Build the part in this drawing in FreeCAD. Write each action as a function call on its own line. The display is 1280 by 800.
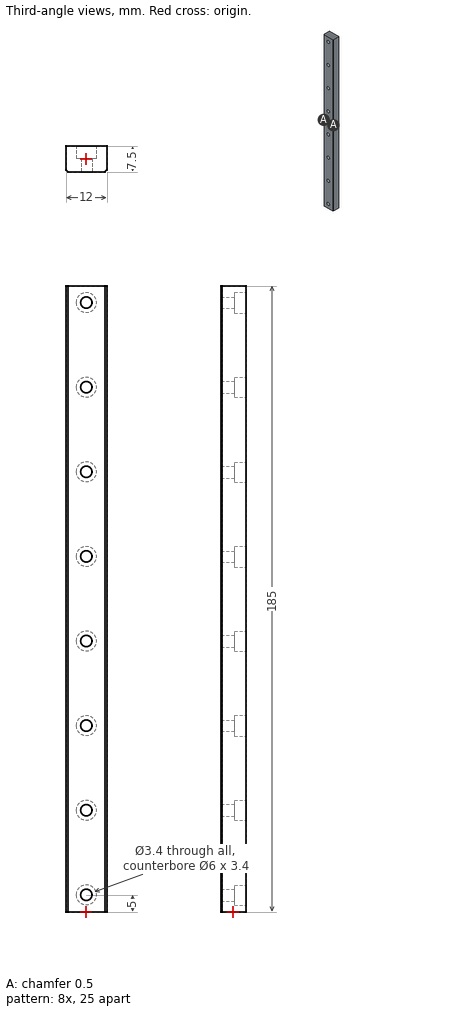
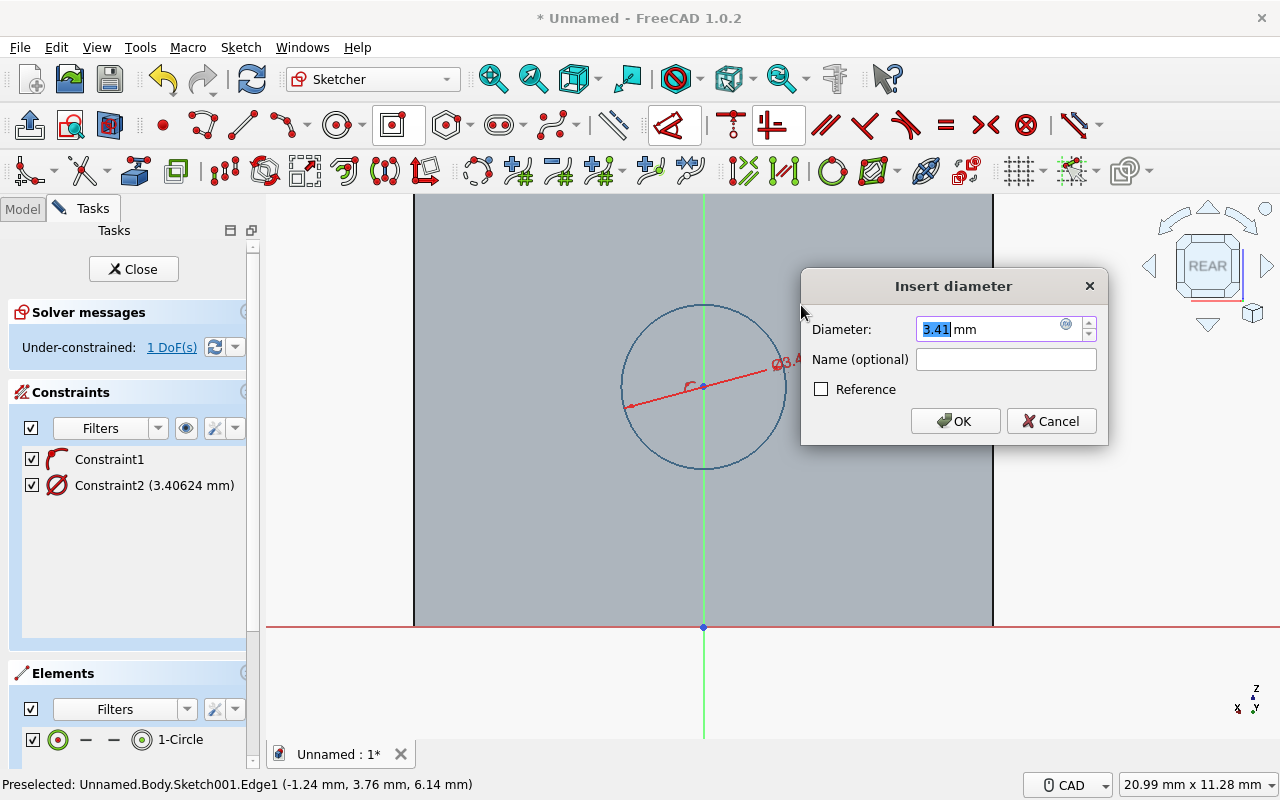
text(3.4)
key(Return)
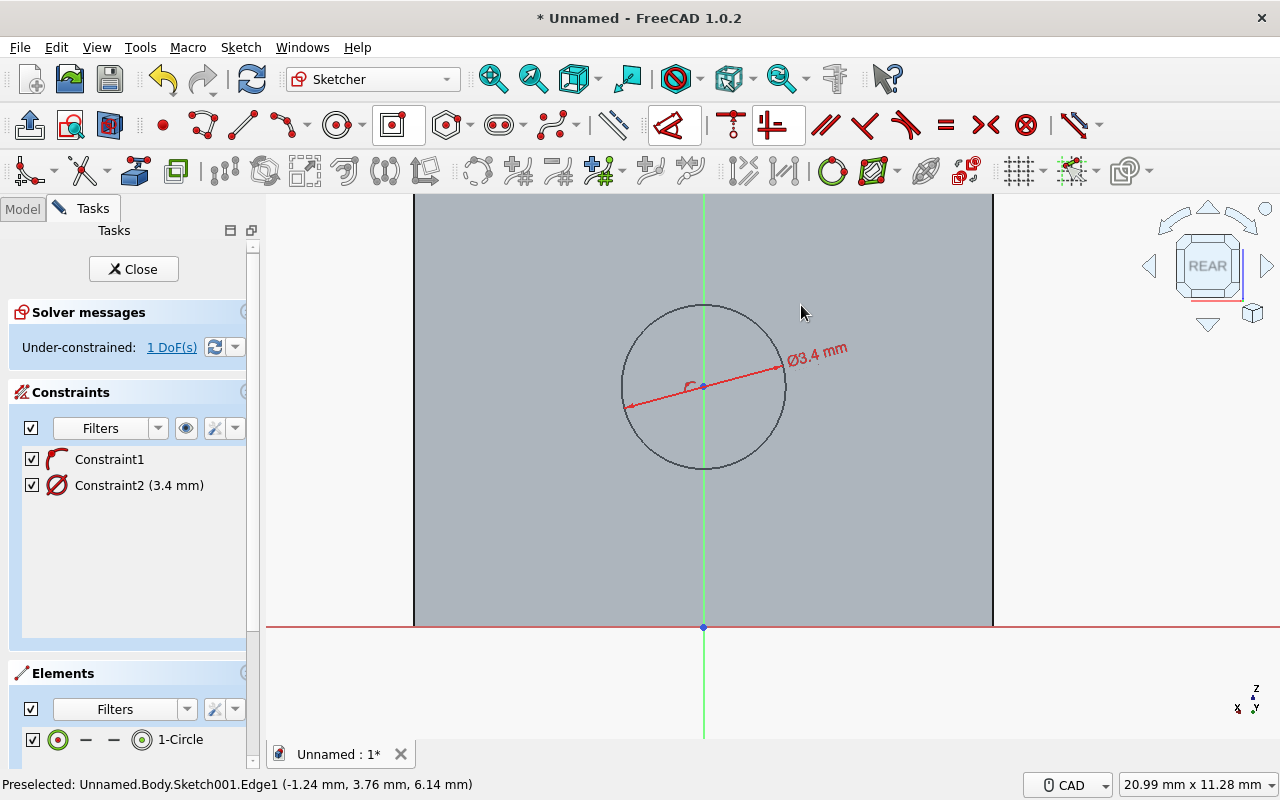
click(704, 387)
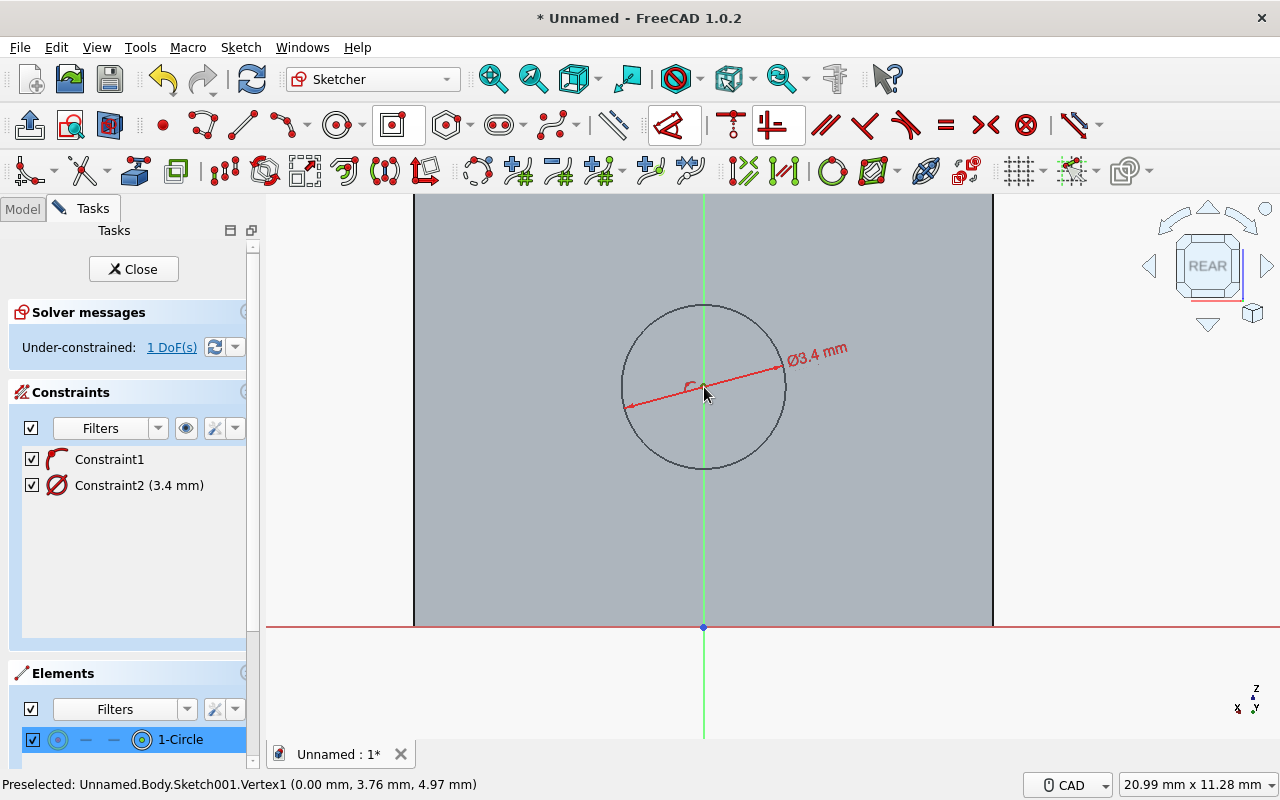
click(696, 126)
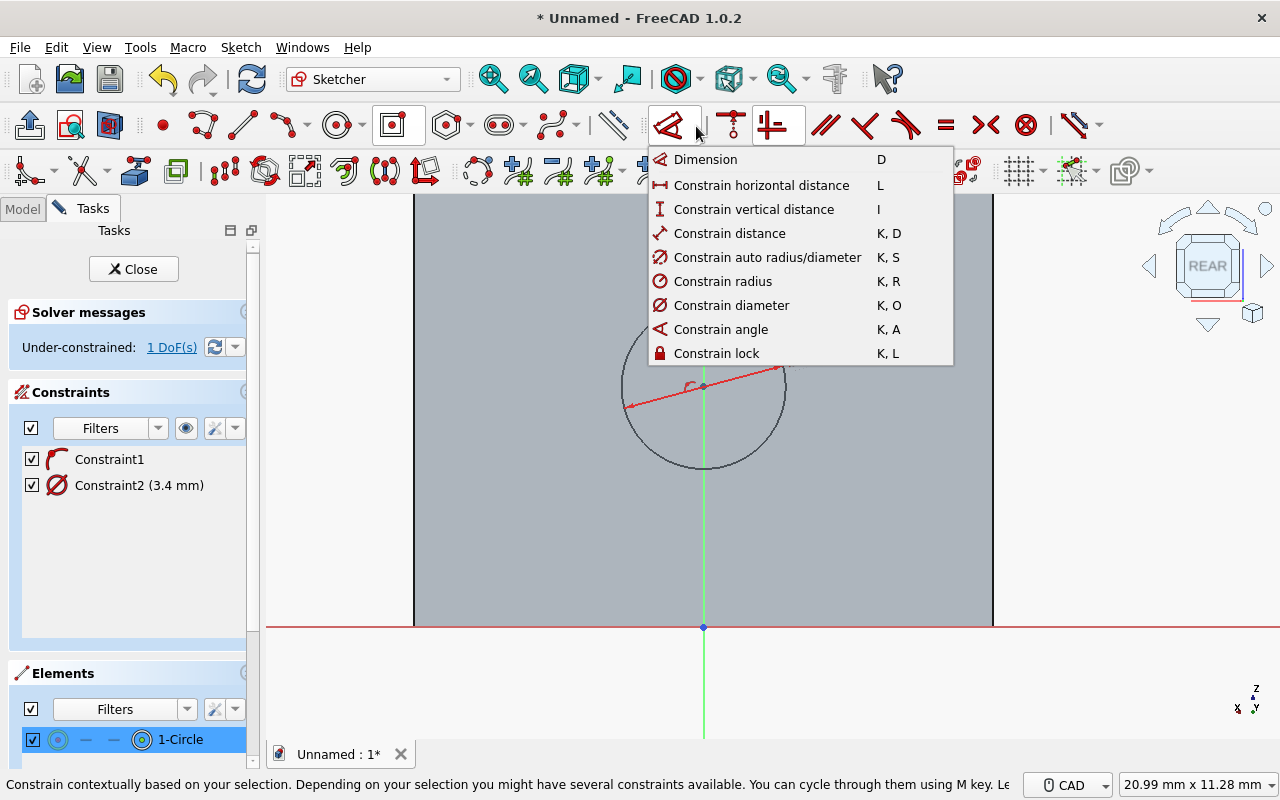
click(801, 209)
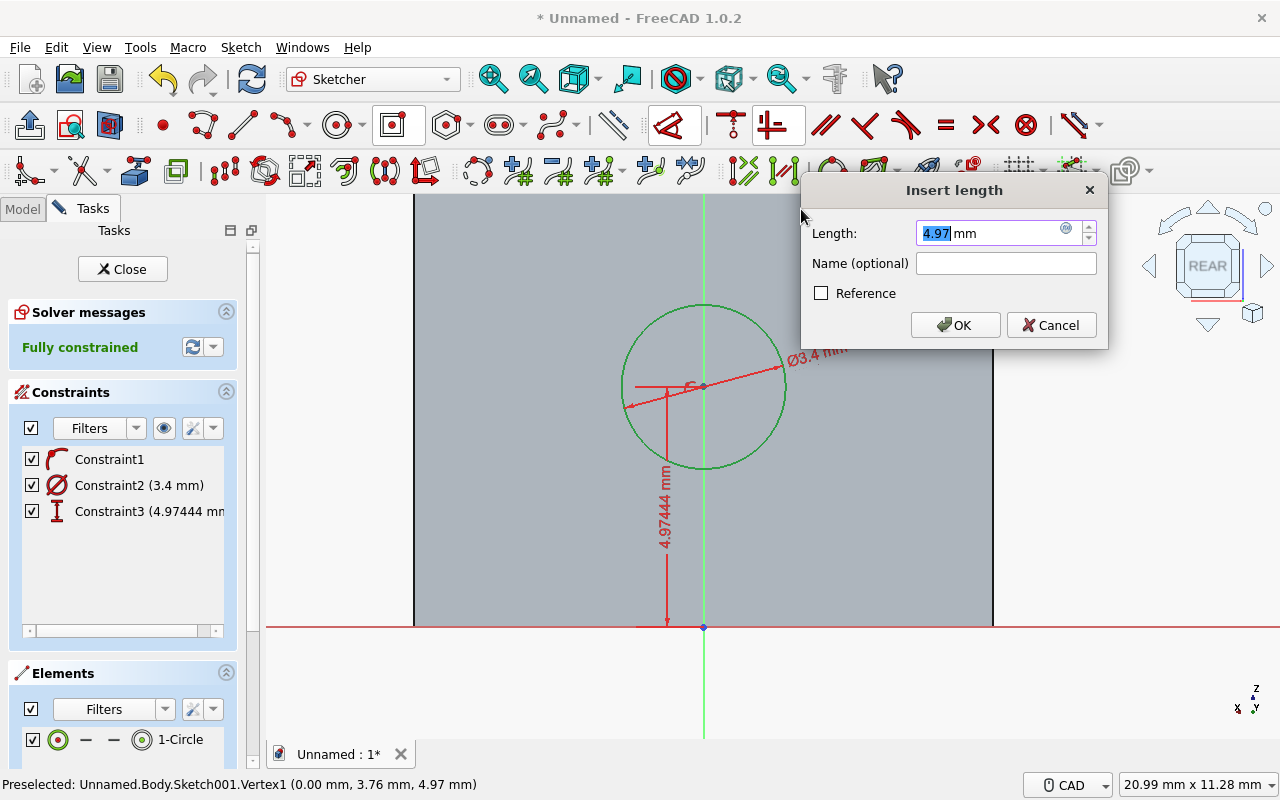
text(5)
key(Return)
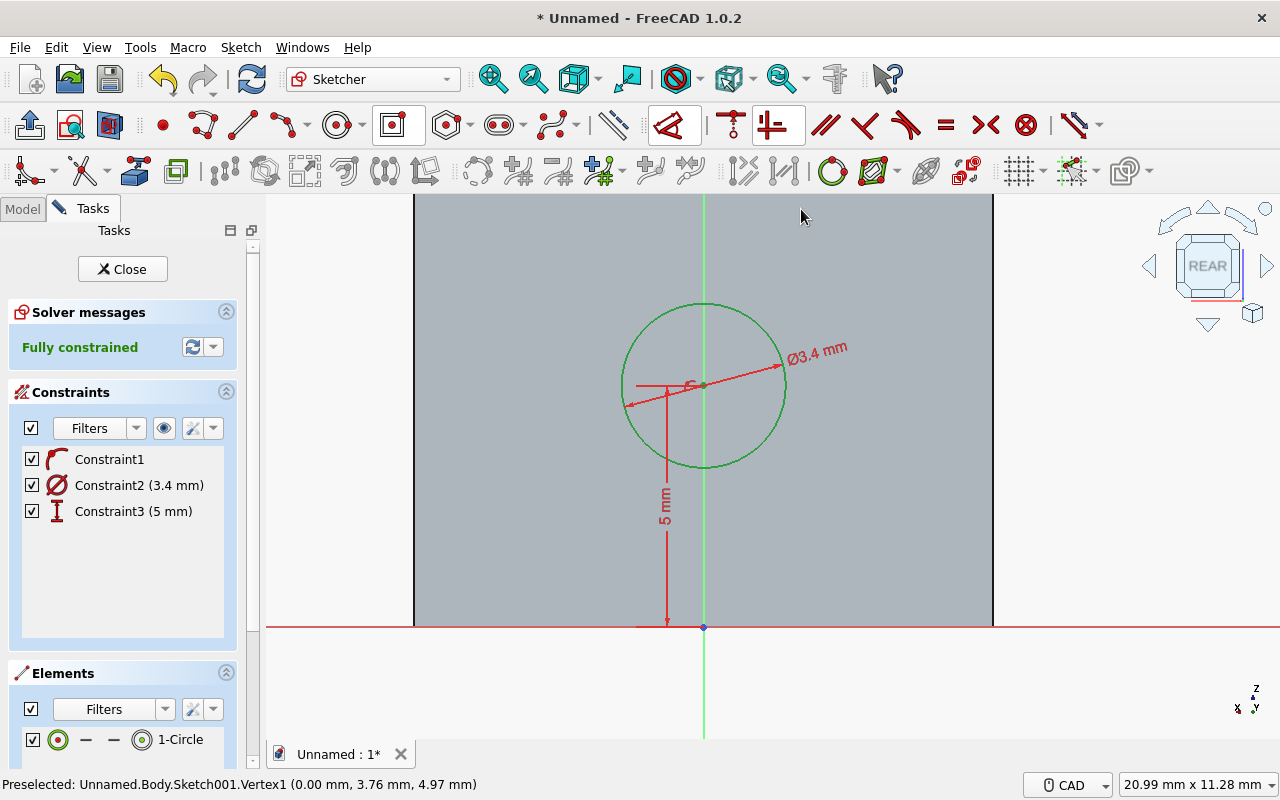
click(123, 269)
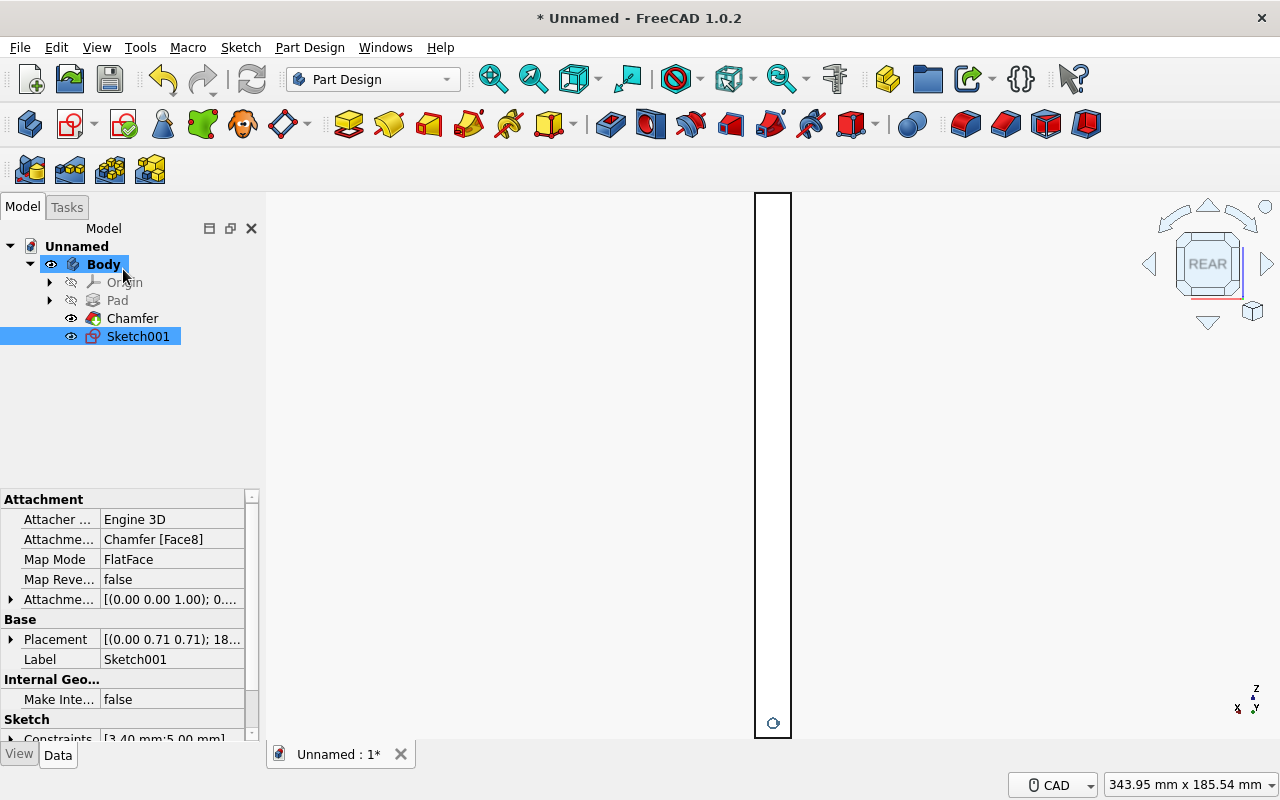
click(652, 124)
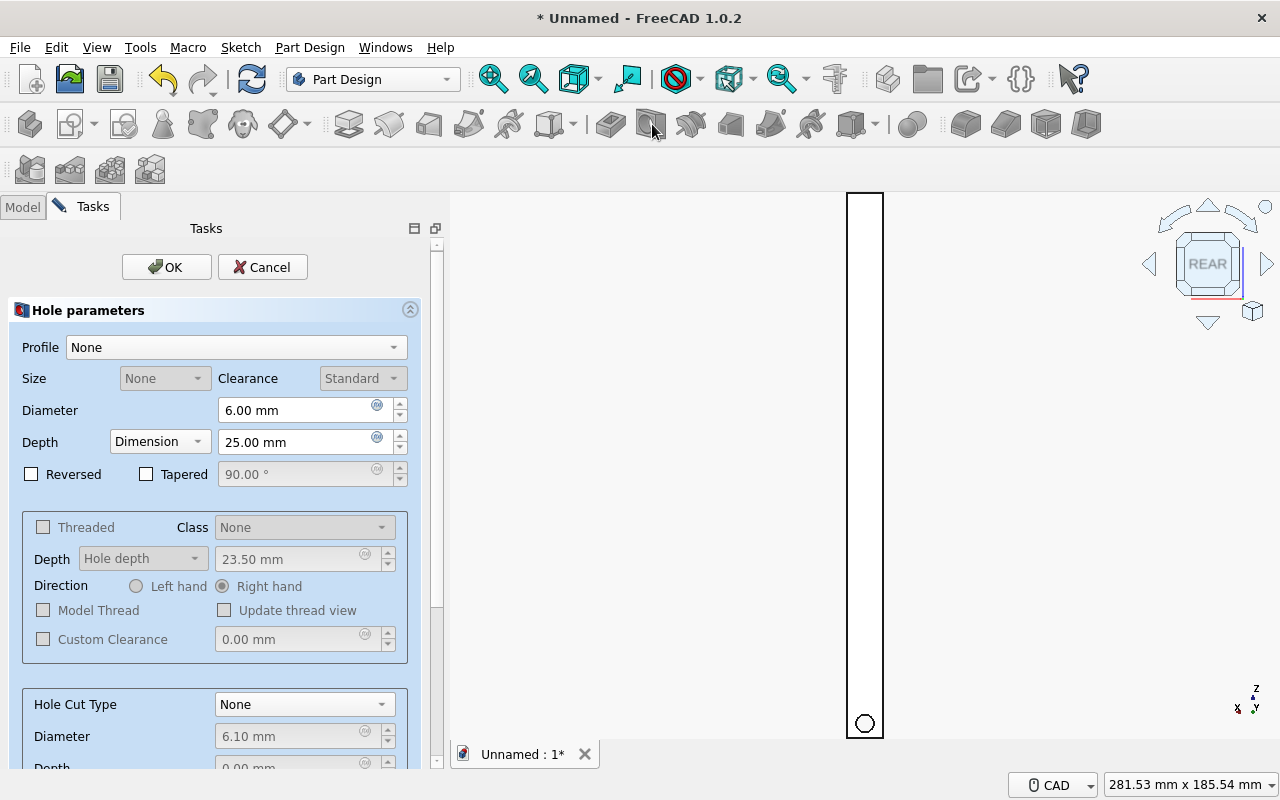
triple_click(305, 410)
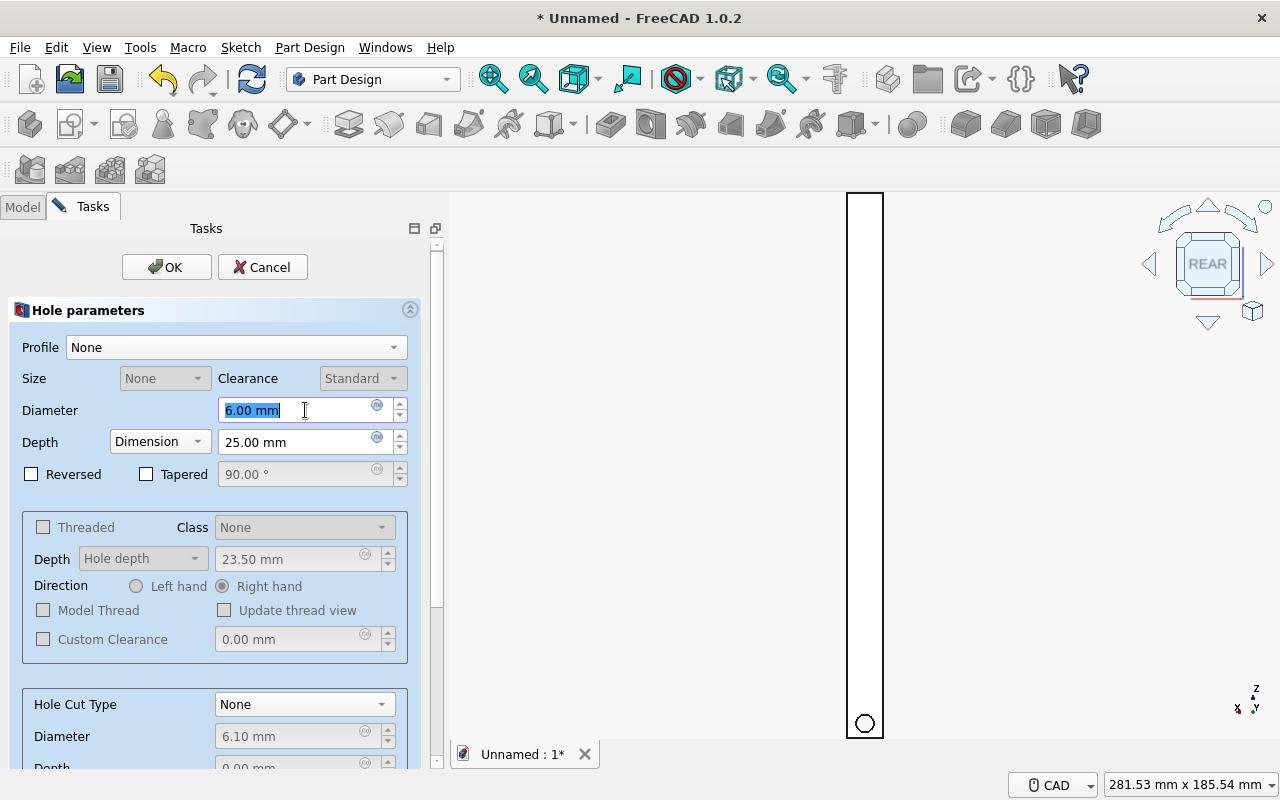
text(3.4)
key(Tab)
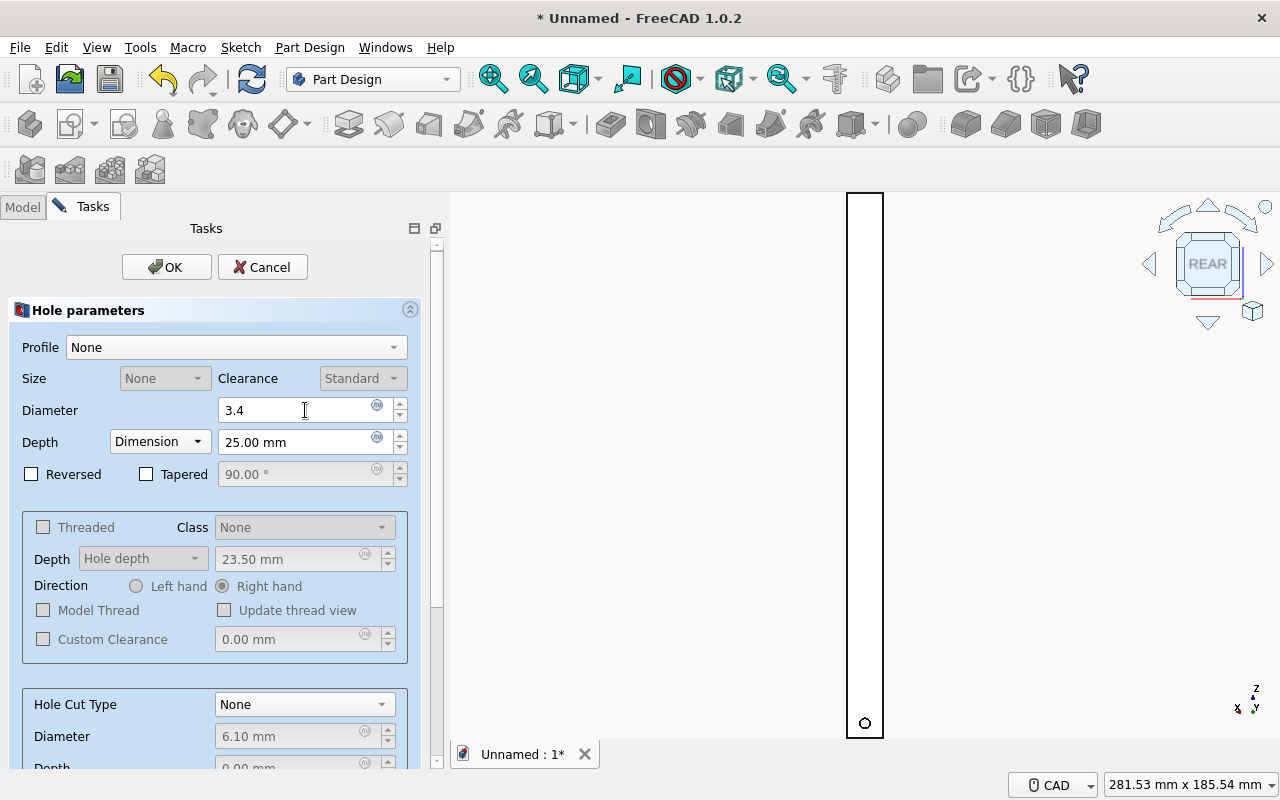
click(161, 442)